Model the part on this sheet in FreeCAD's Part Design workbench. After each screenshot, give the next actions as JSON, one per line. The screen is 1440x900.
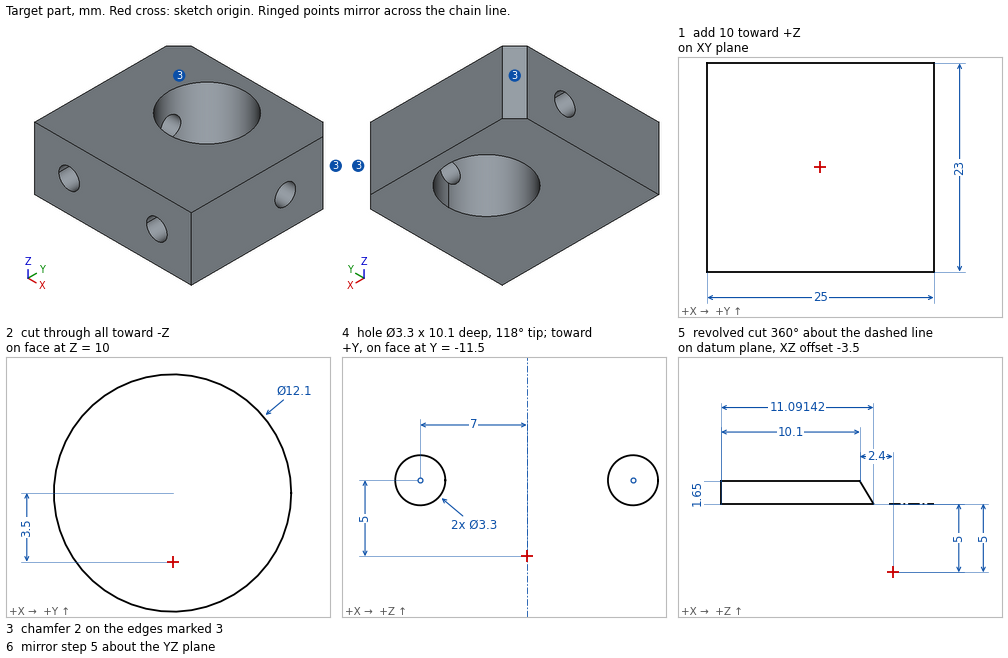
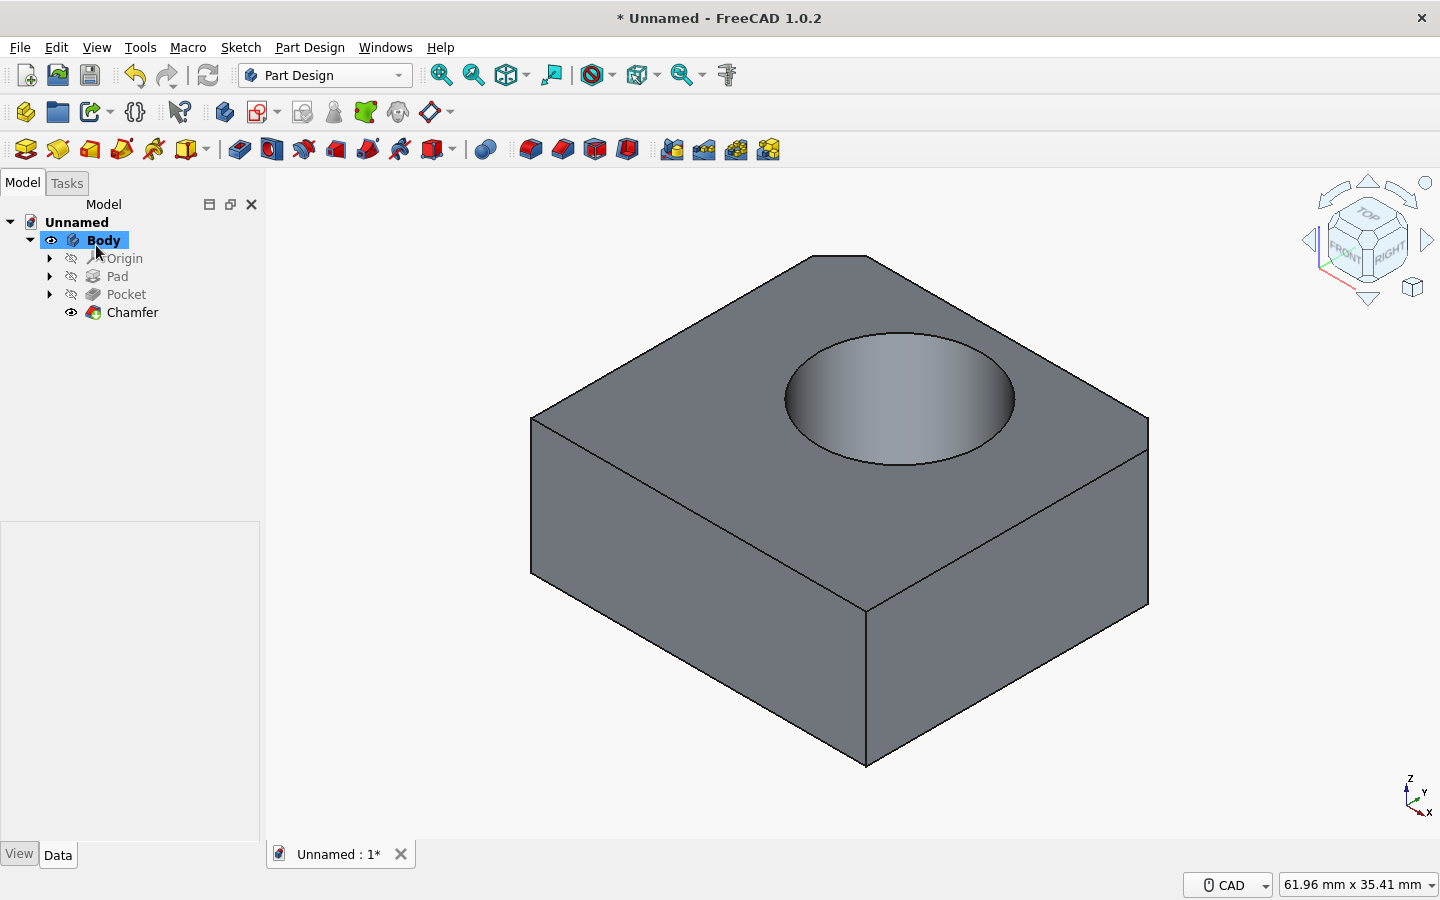
{"action": "left_click", "coordinate": [795, 647]}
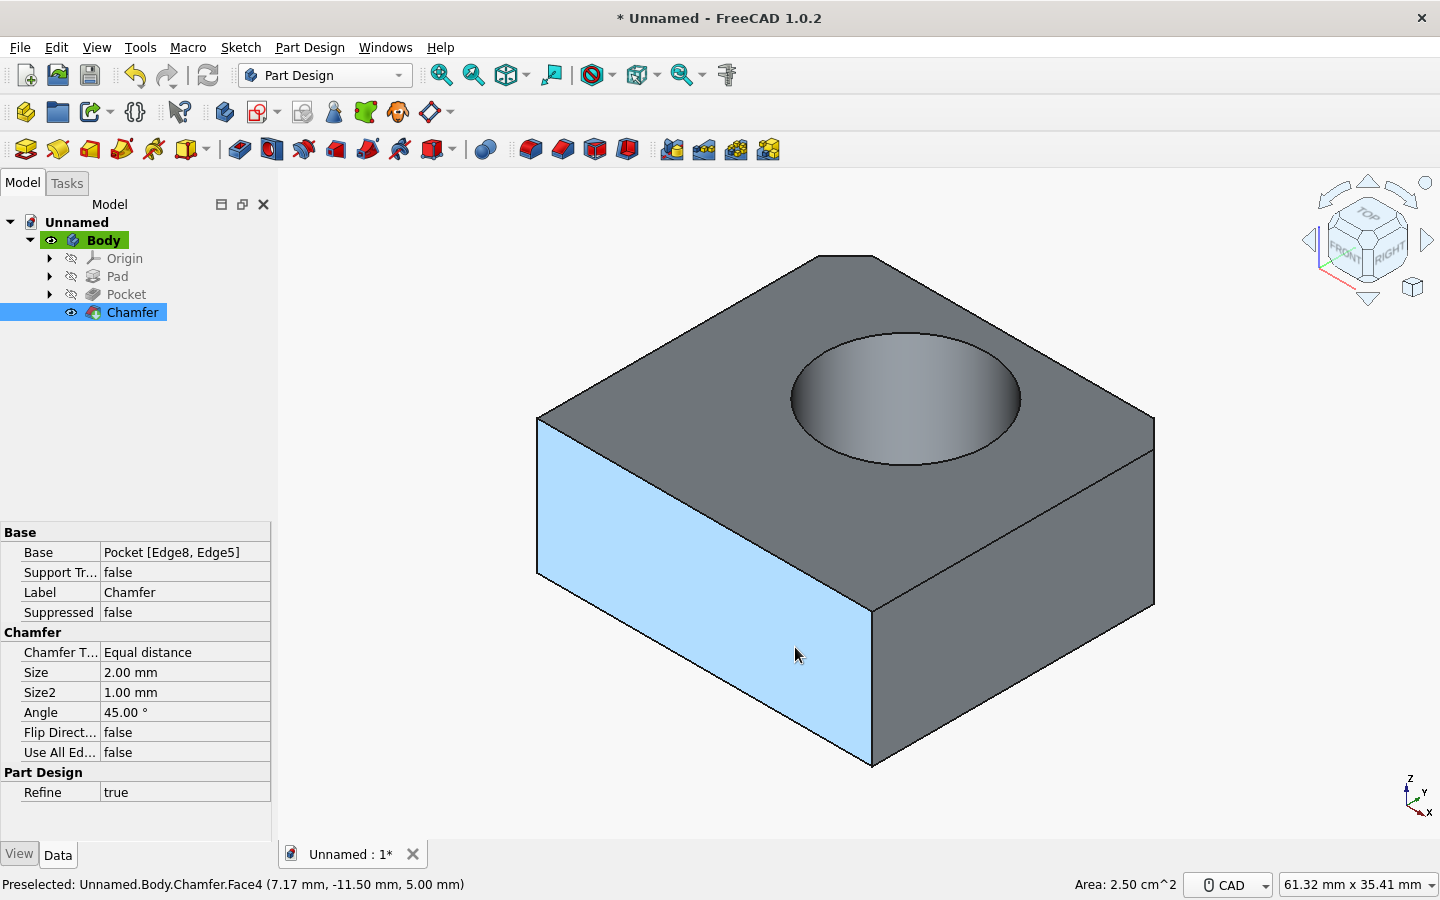
{"action": "left_click", "coordinate": [258, 112]}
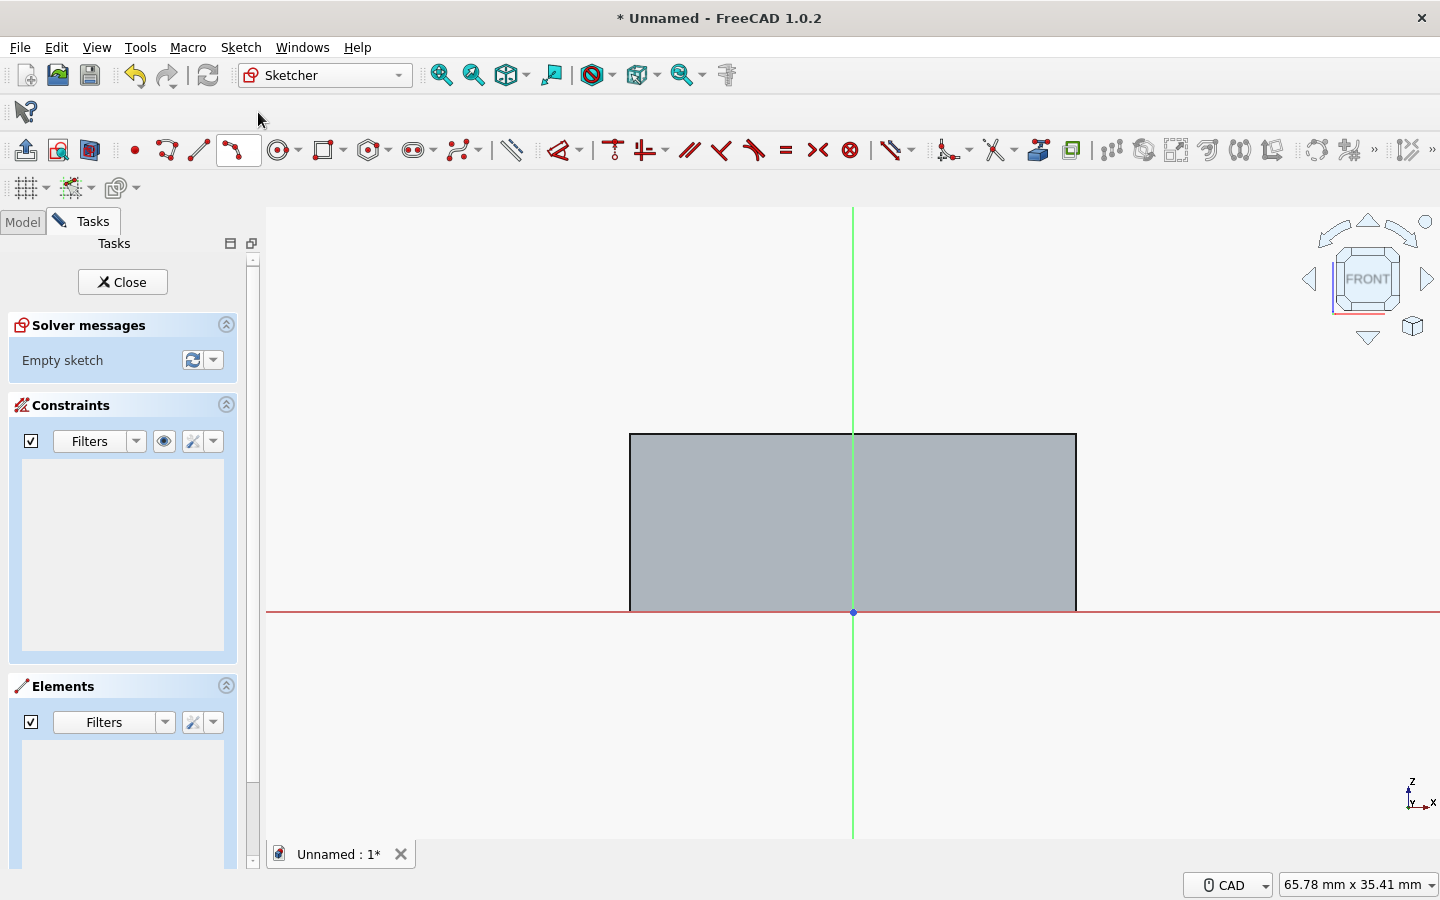
{"action": "scroll", "coordinate": [909, 577], "scroll_direction": "up", "scroll_amount": 4}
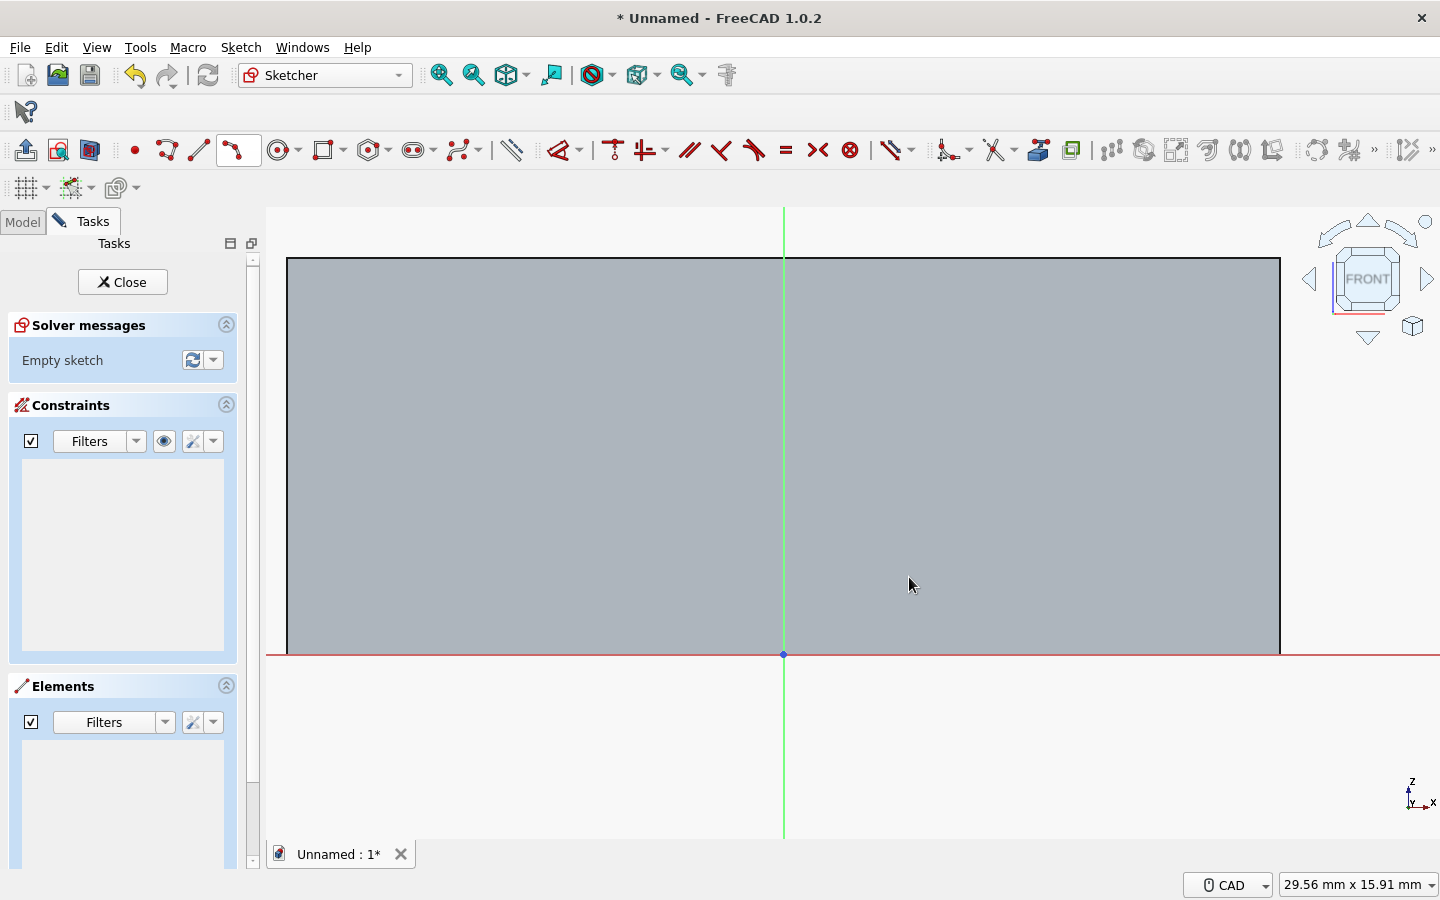
{"action": "left_click", "coordinate": [278, 150]}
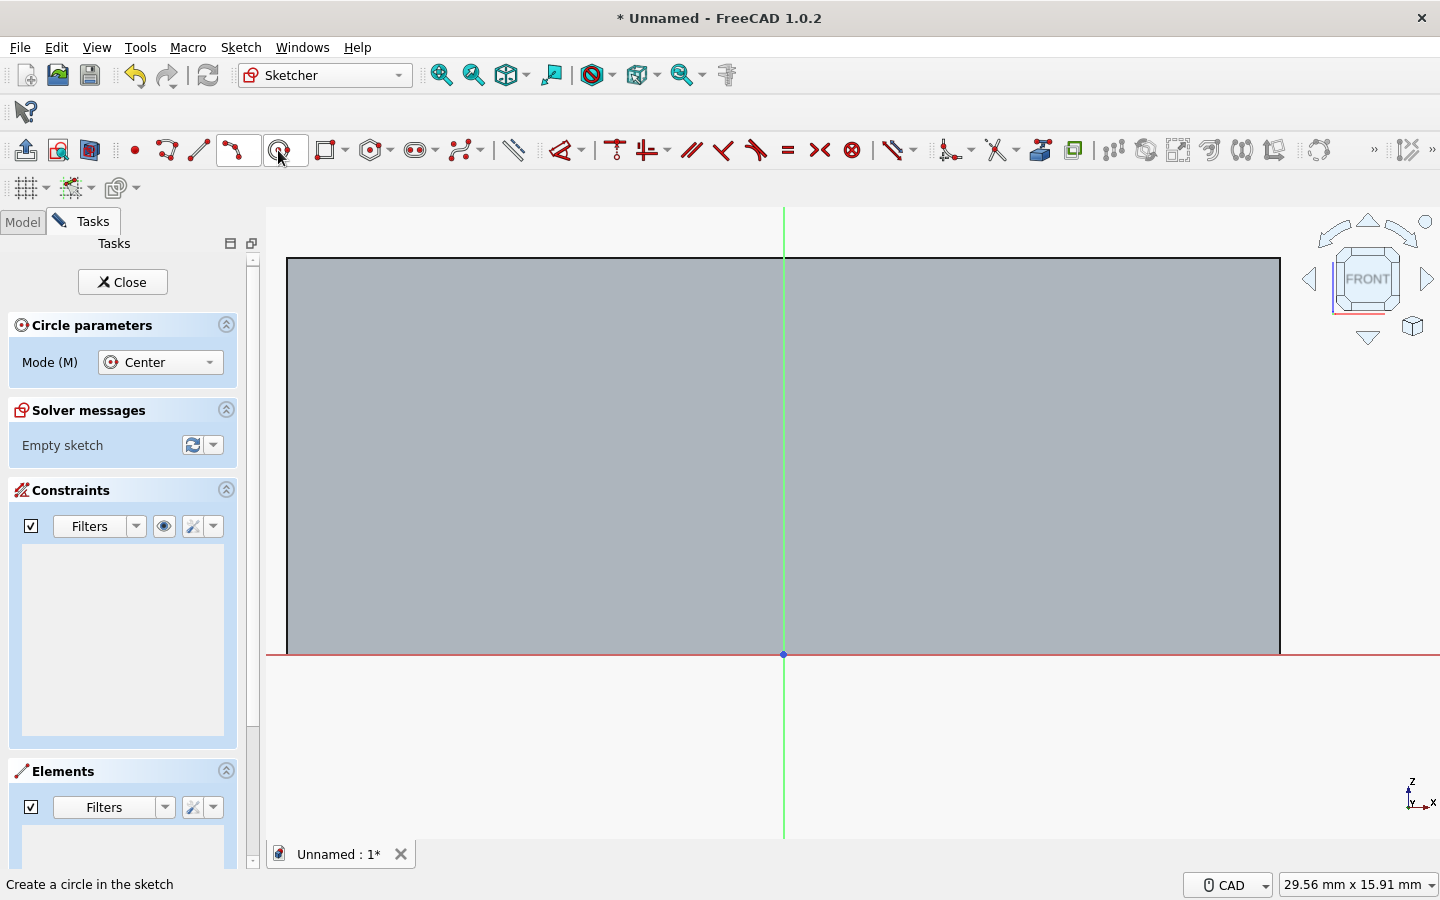
{"action": "left_click", "coordinate": [506, 456]}
{"action": "left_click", "coordinate": [552, 410]}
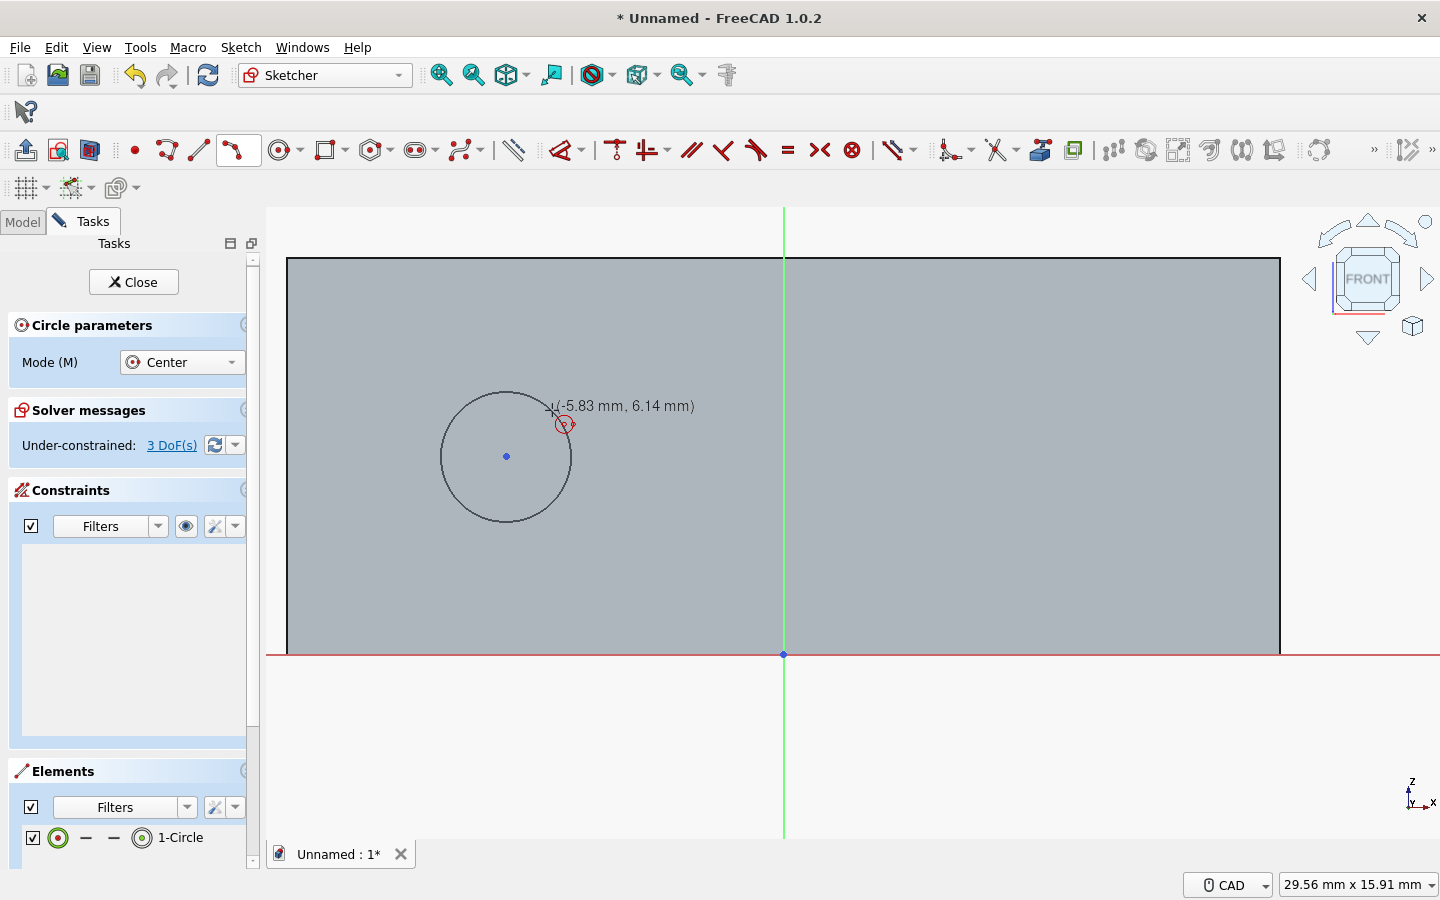
{"action": "left_click", "coordinate": [1062, 456]}
{"action": "left_click", "coordinate": [1108, 410]}
{"action": "key", "text": "Escape"}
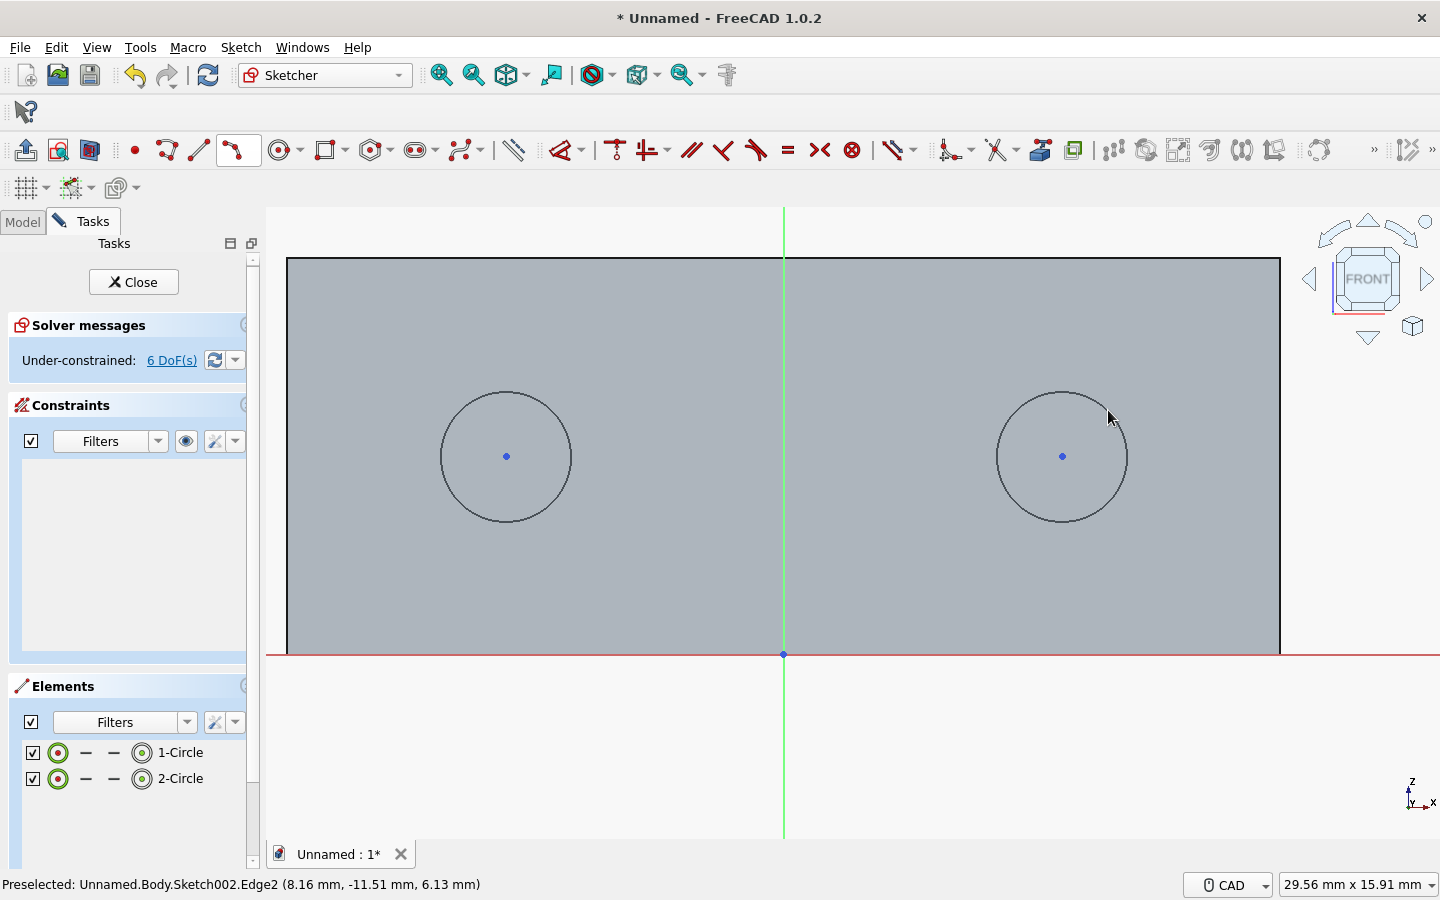
{"action": "left_click", "coordinate": [552, 411]}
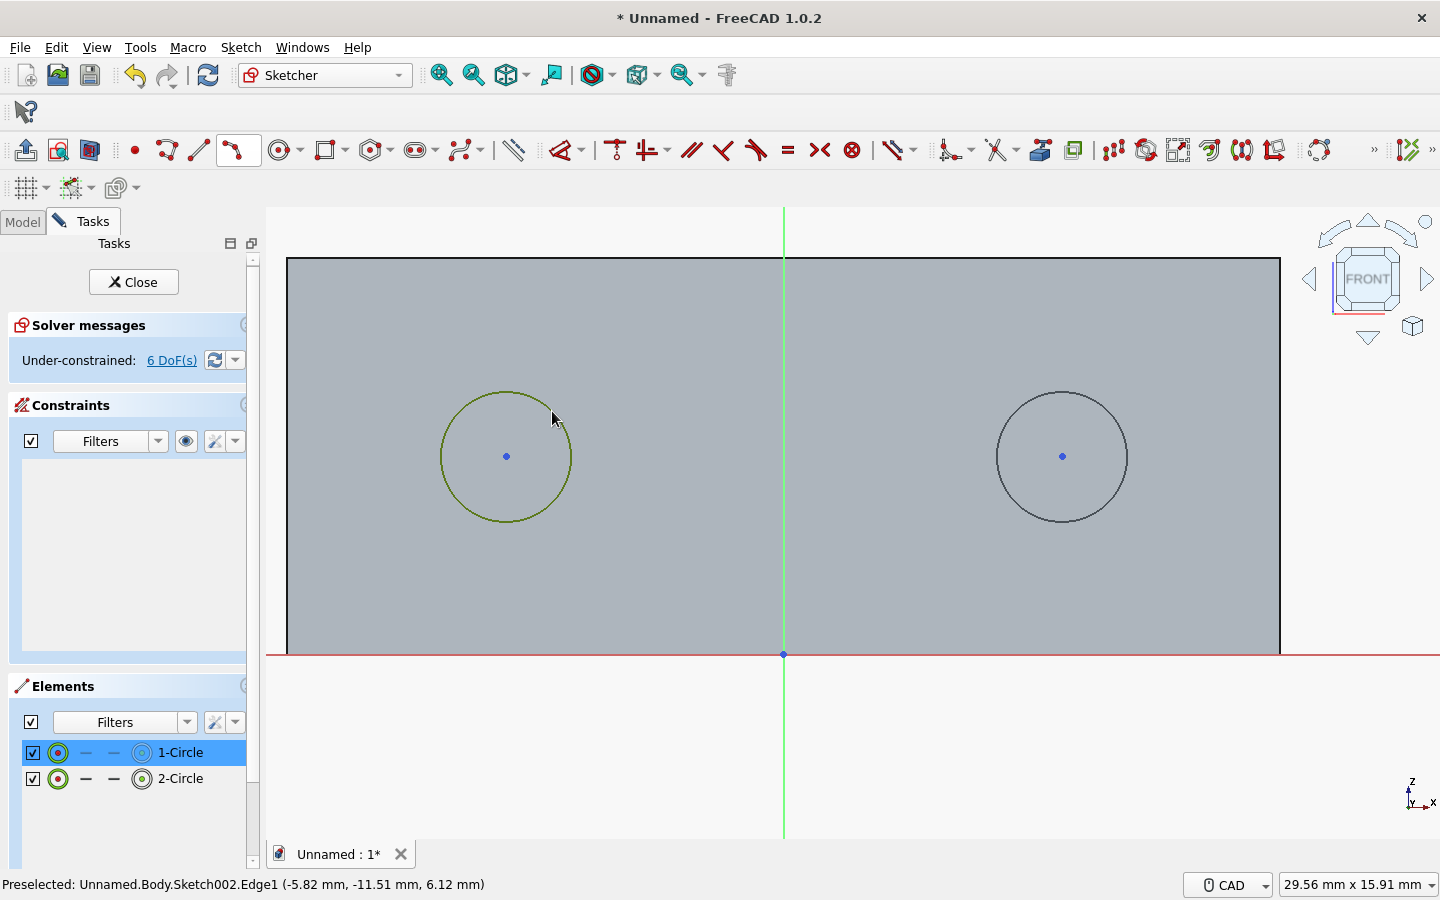
{"action": "left_click", "coordinate": [1108, 411]}